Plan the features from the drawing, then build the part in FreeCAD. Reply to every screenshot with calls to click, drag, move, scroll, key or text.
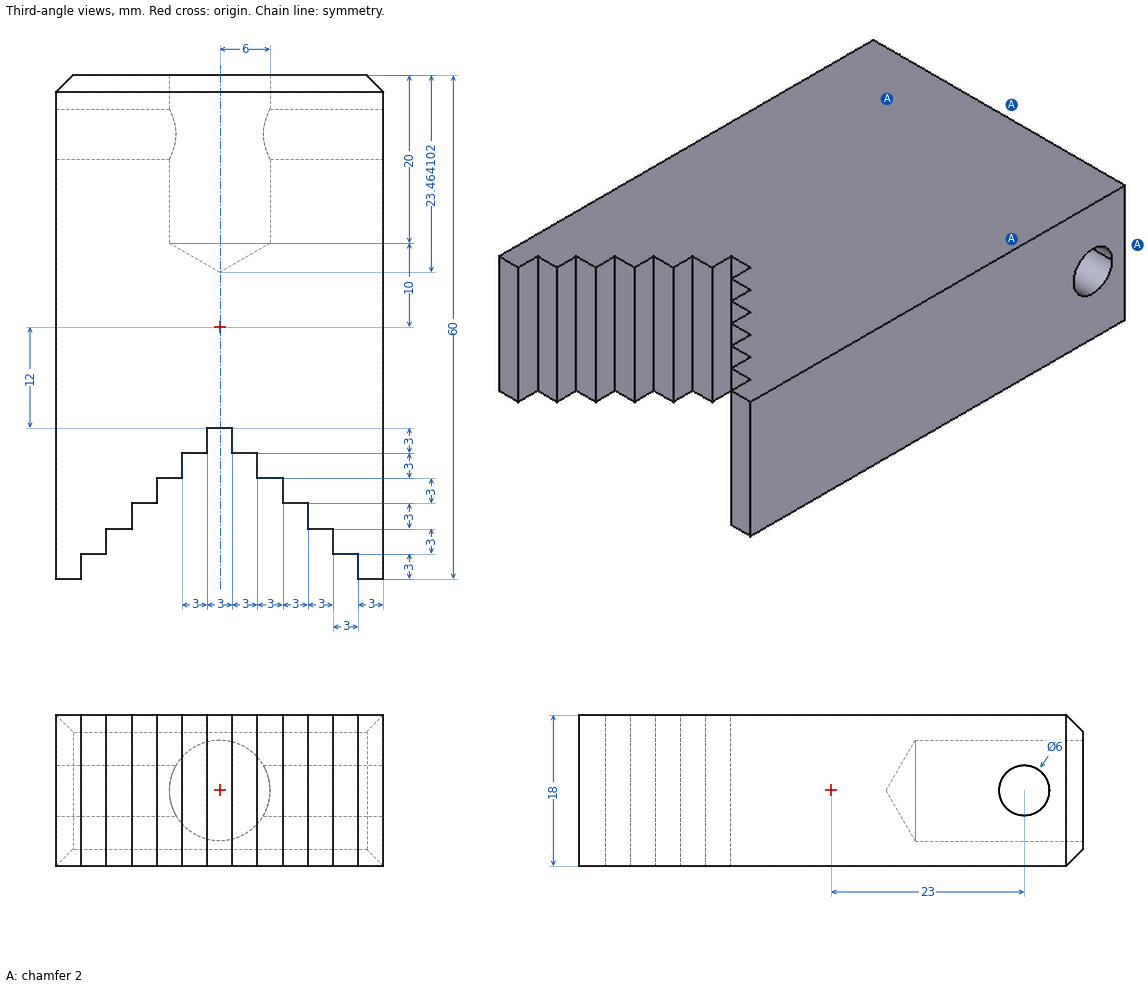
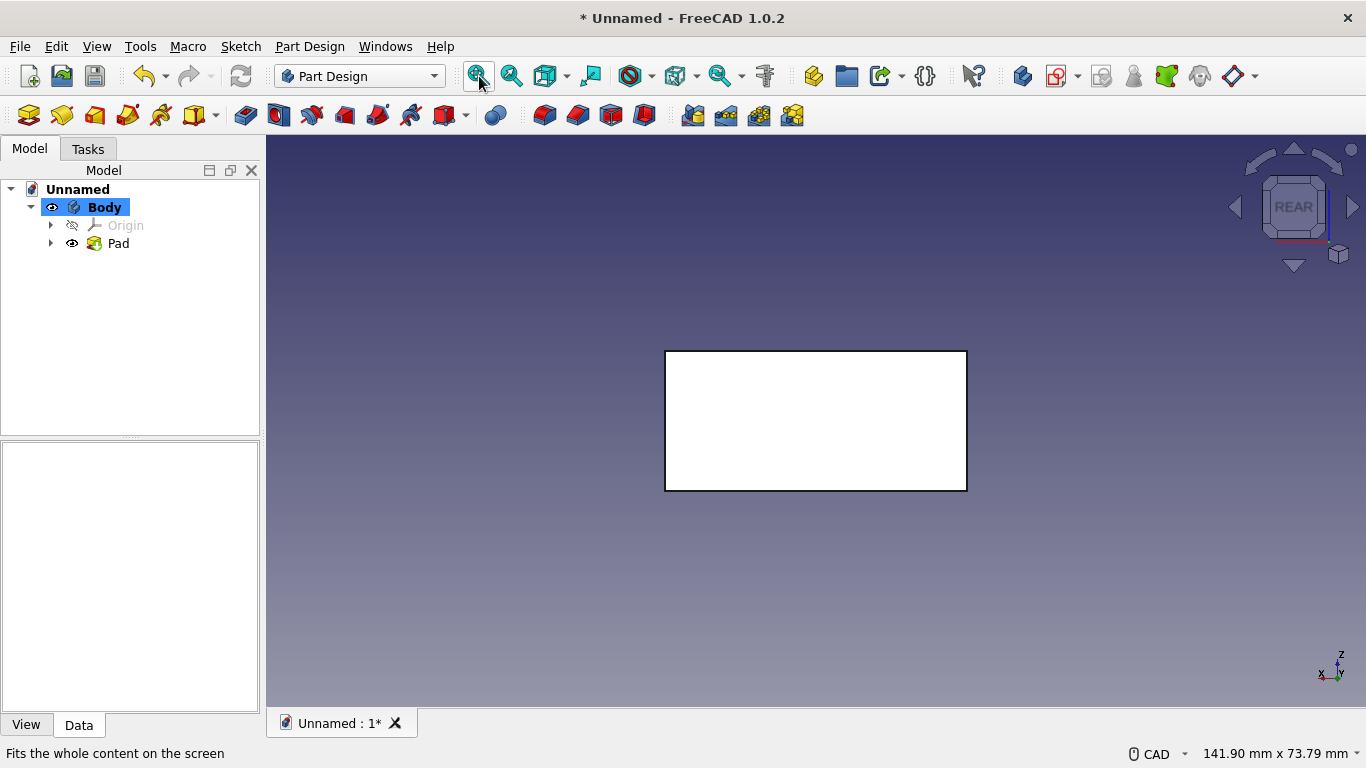
click(773, 420)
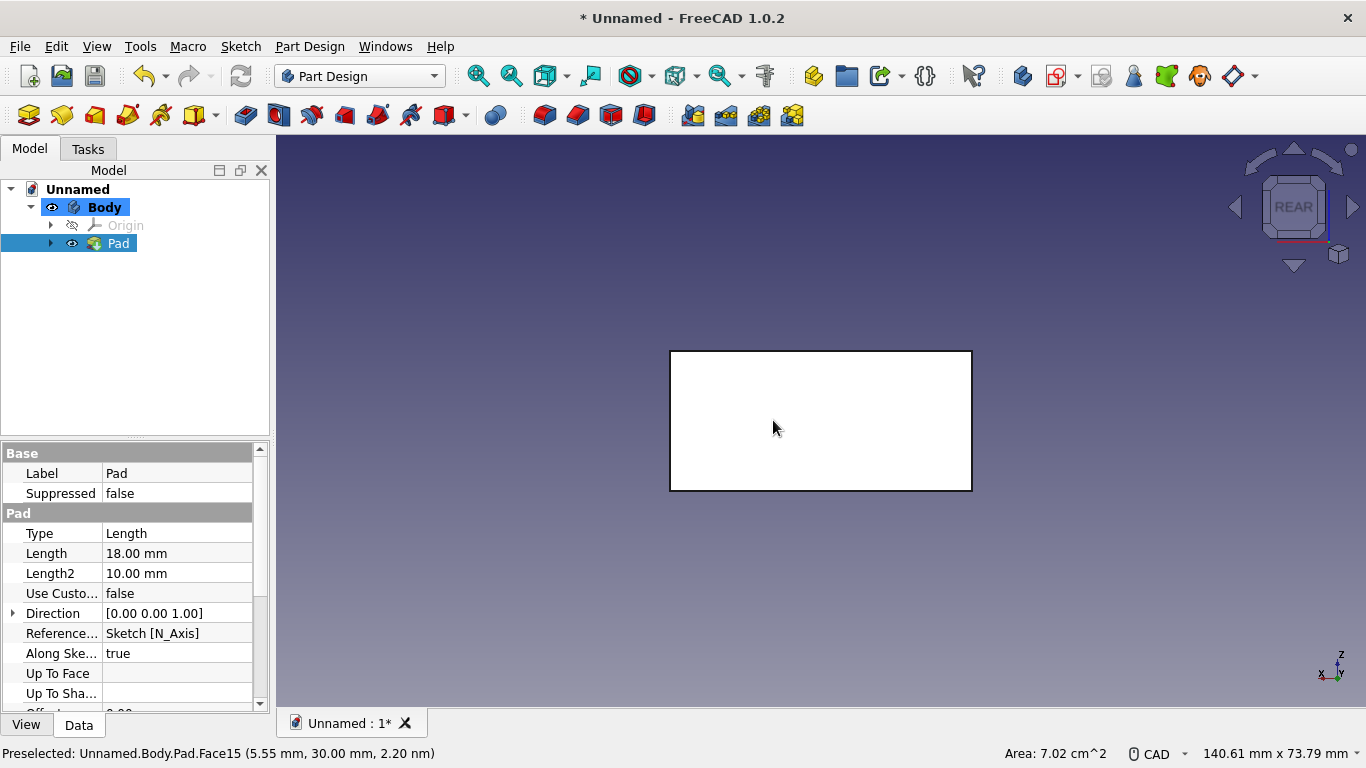
click(578, 116)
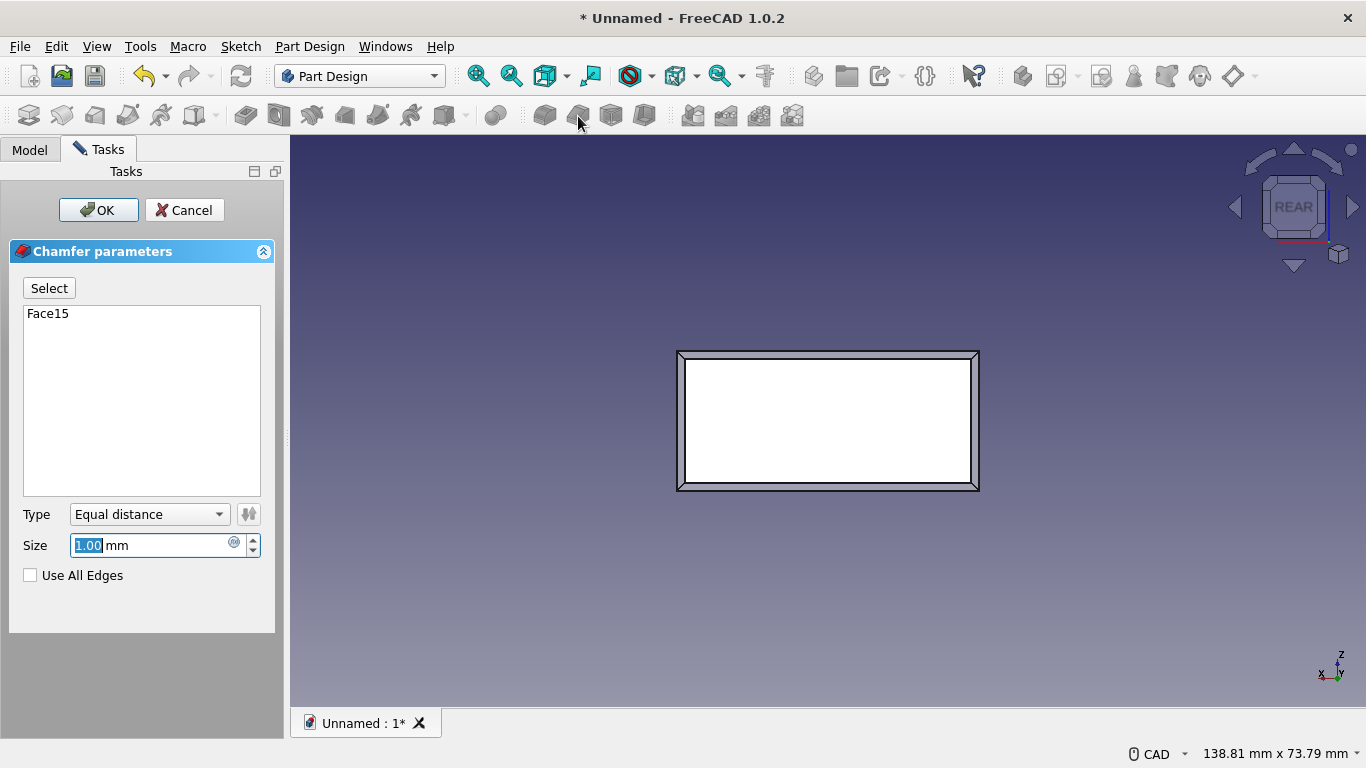
text(2)
key(Tab)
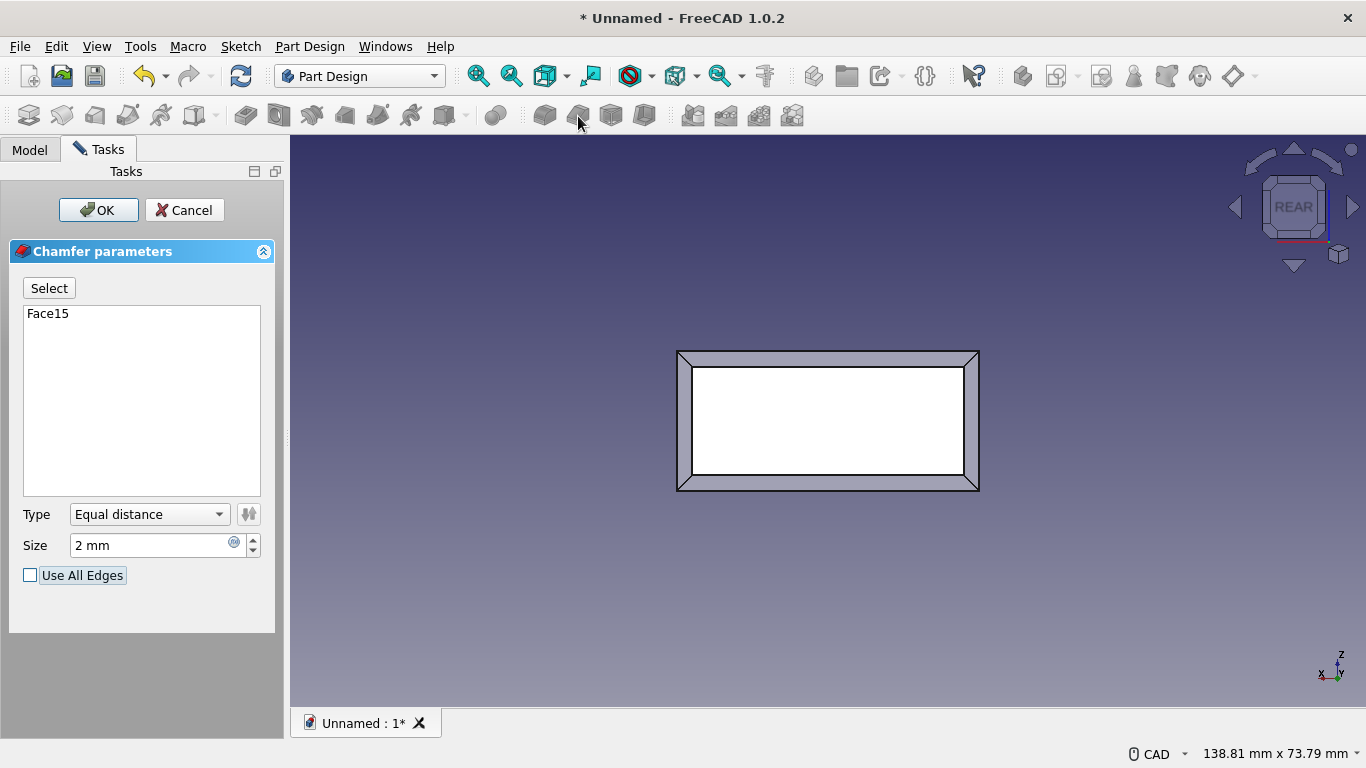
click(99, 210)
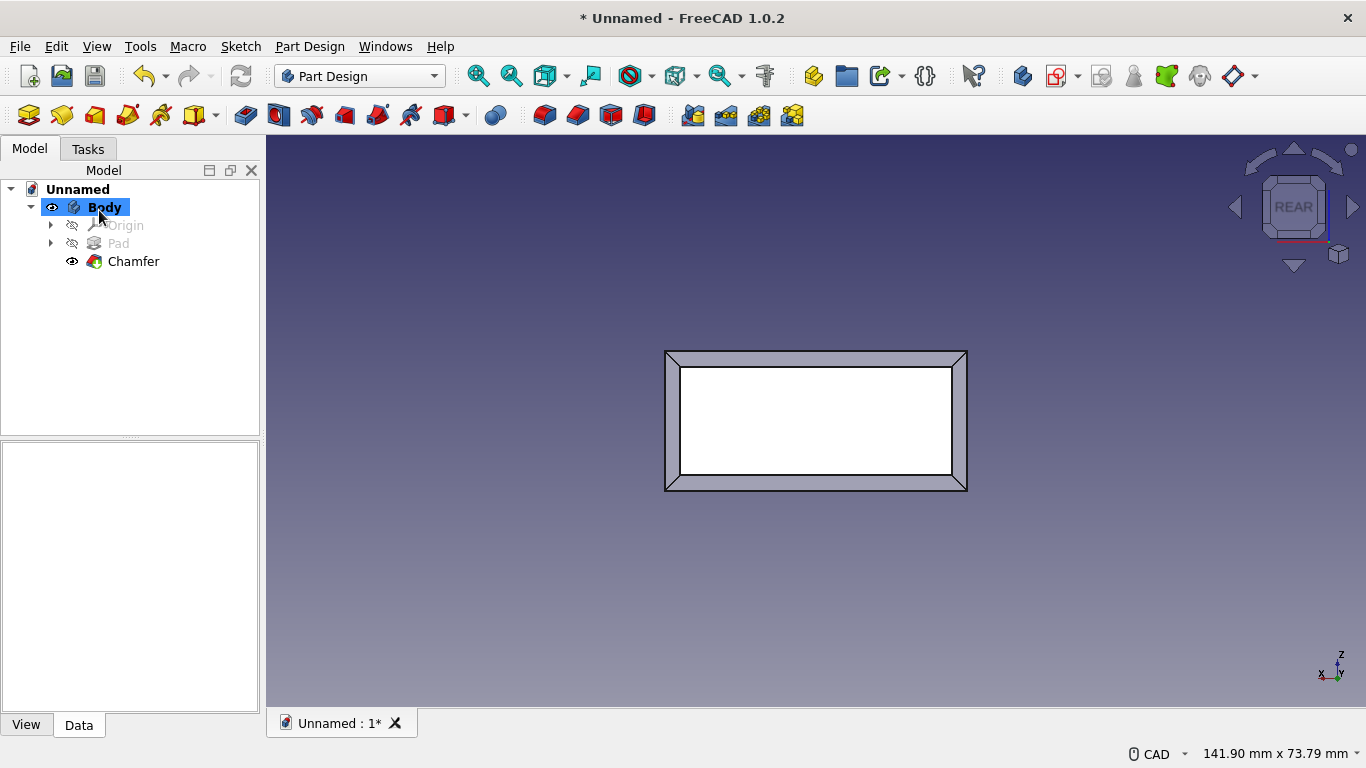
click(479, 76)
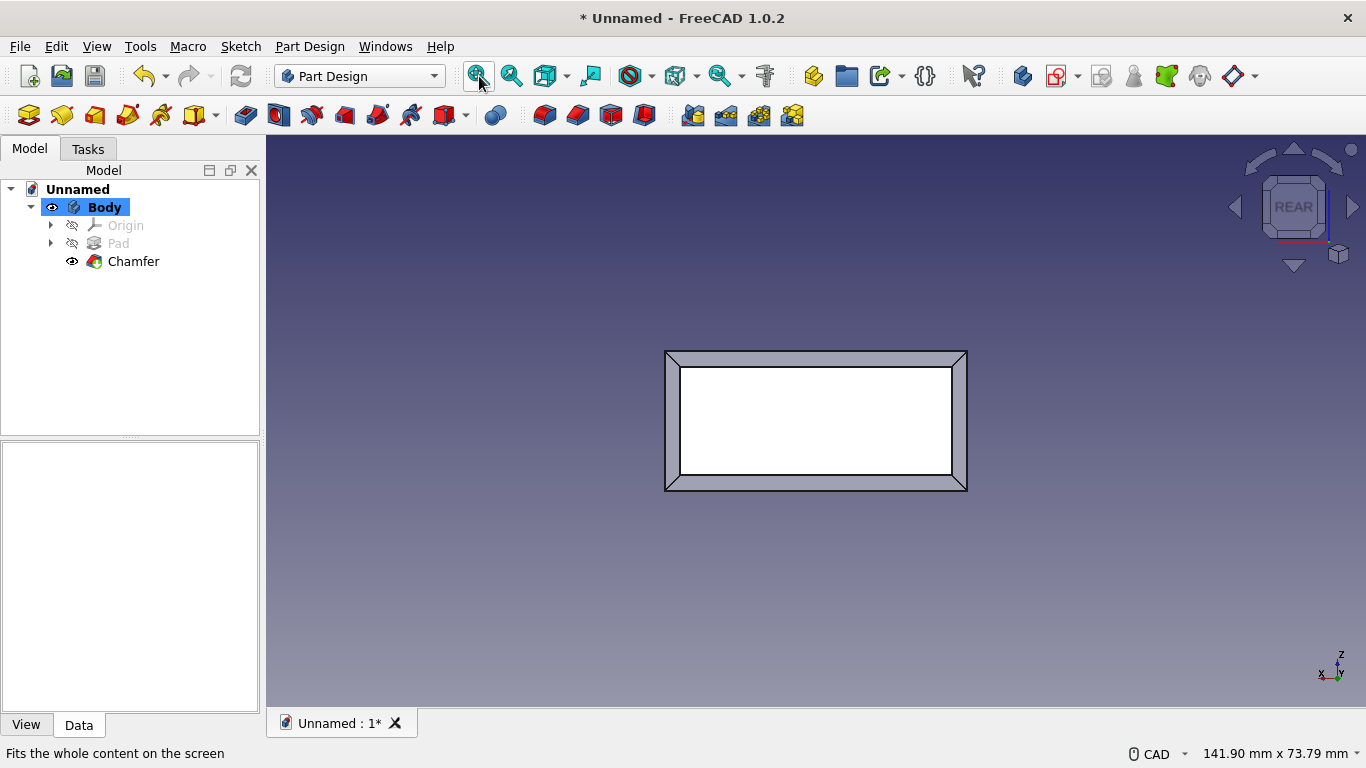
key(0)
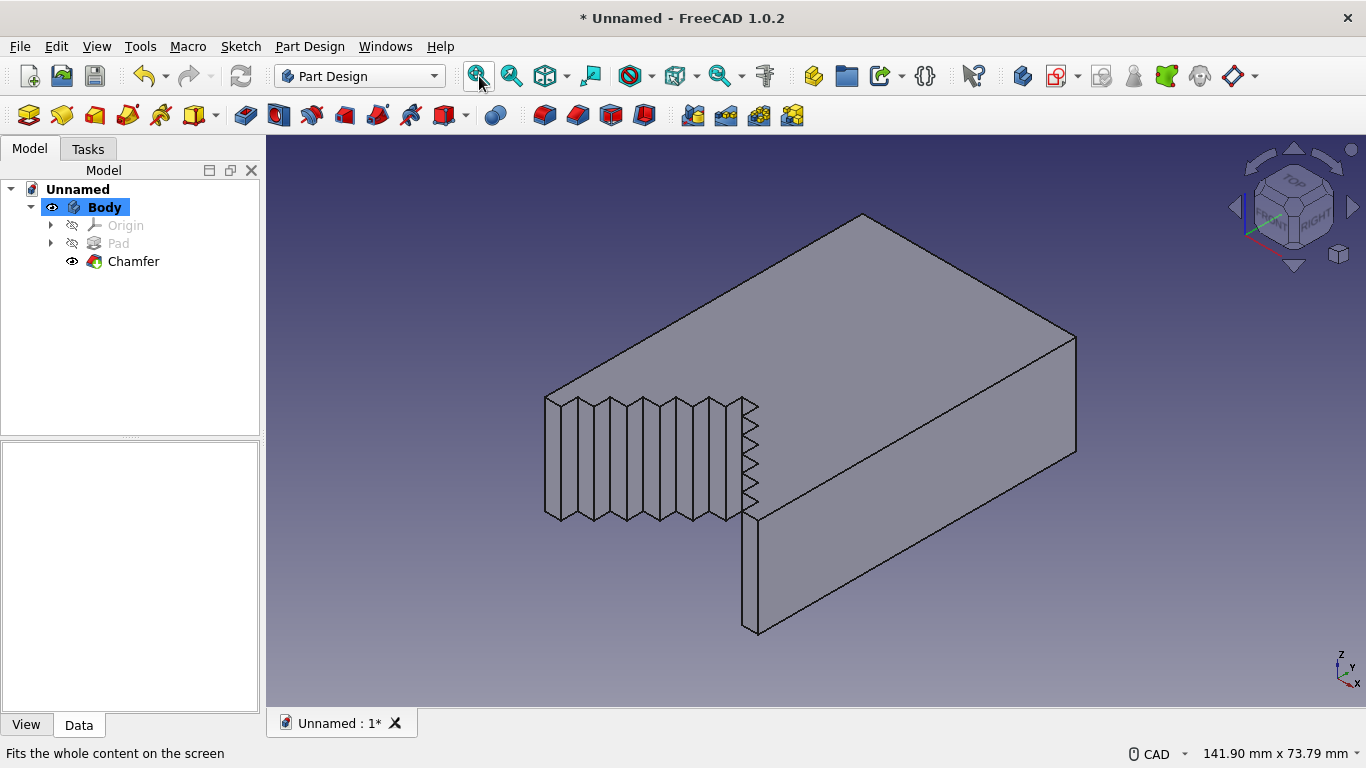
click(1008, 432)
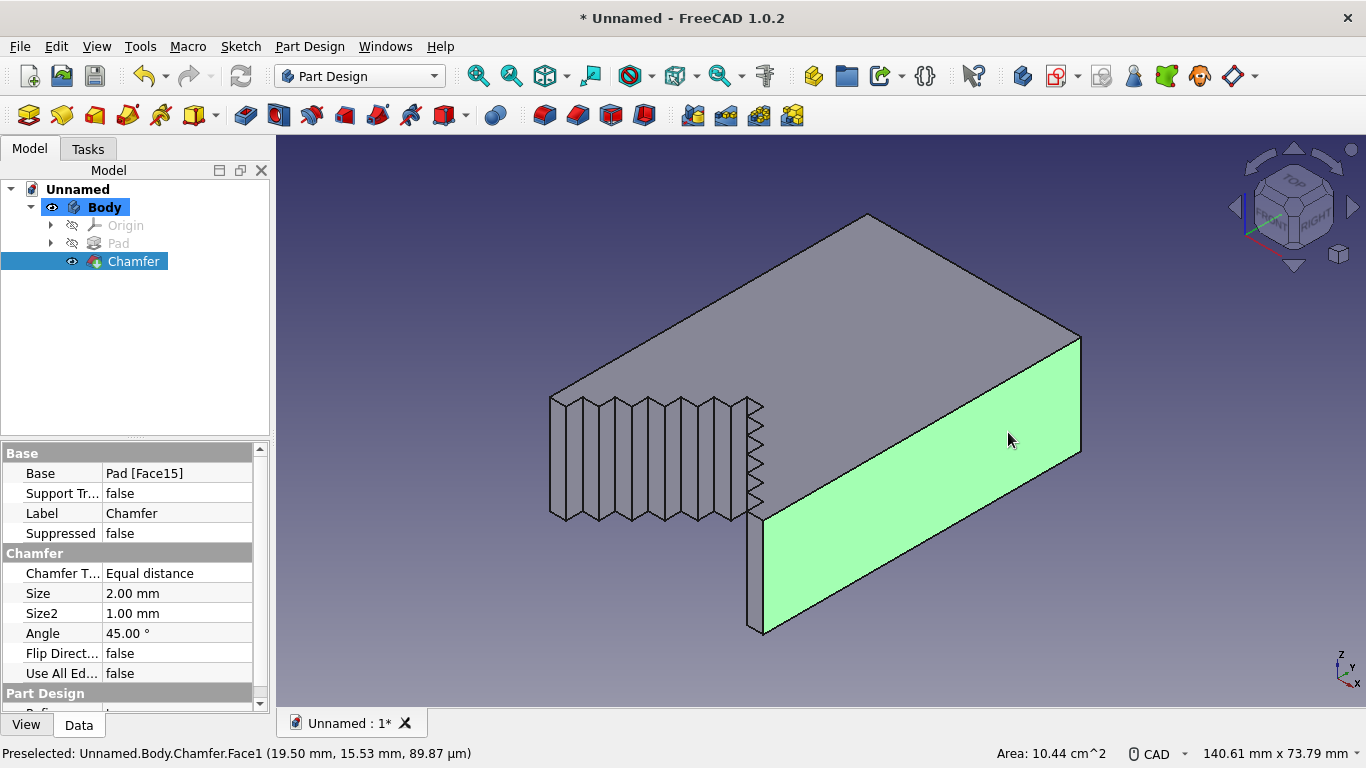
click(1056, 76)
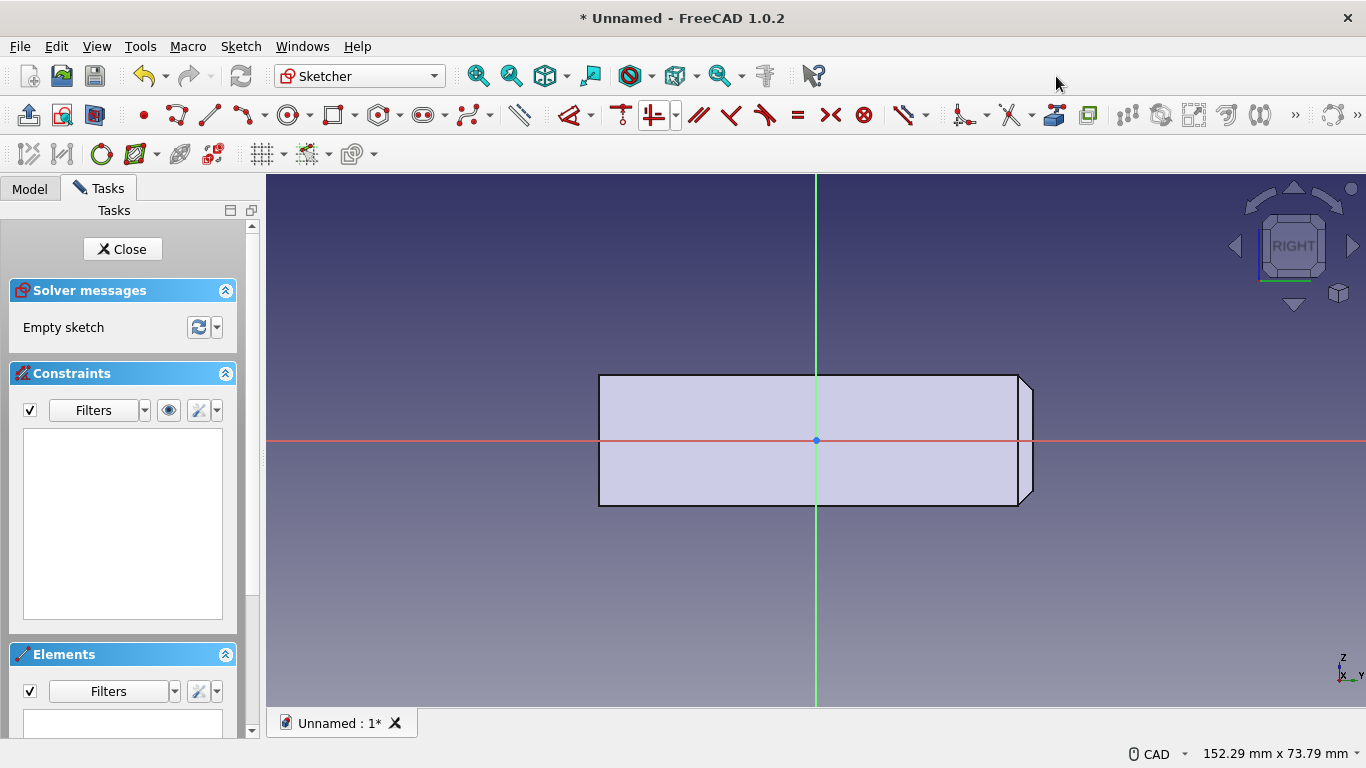
scroll(1019, 440, up, 10)